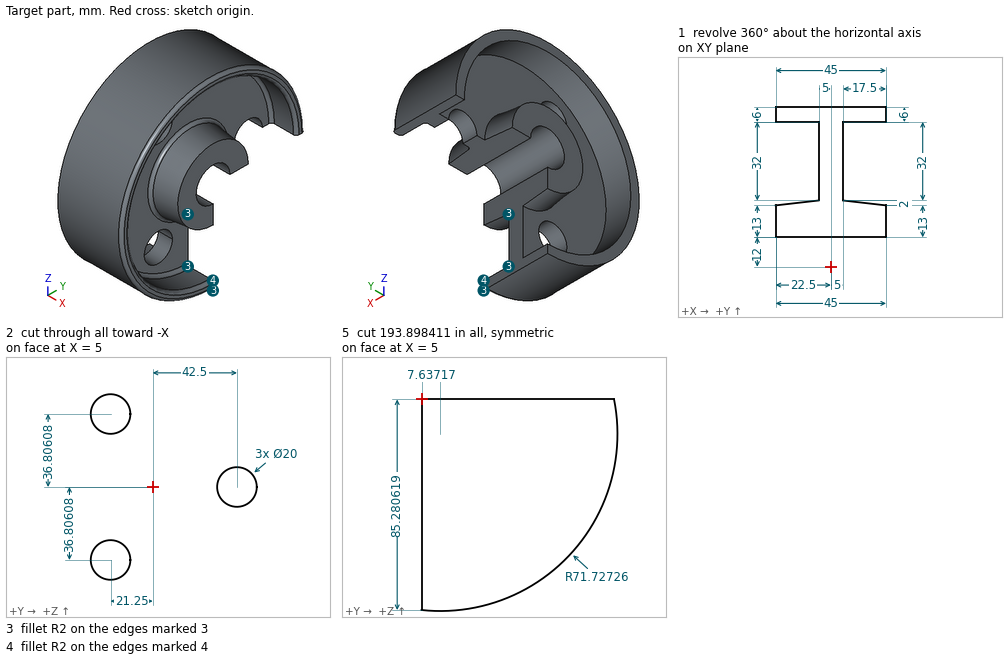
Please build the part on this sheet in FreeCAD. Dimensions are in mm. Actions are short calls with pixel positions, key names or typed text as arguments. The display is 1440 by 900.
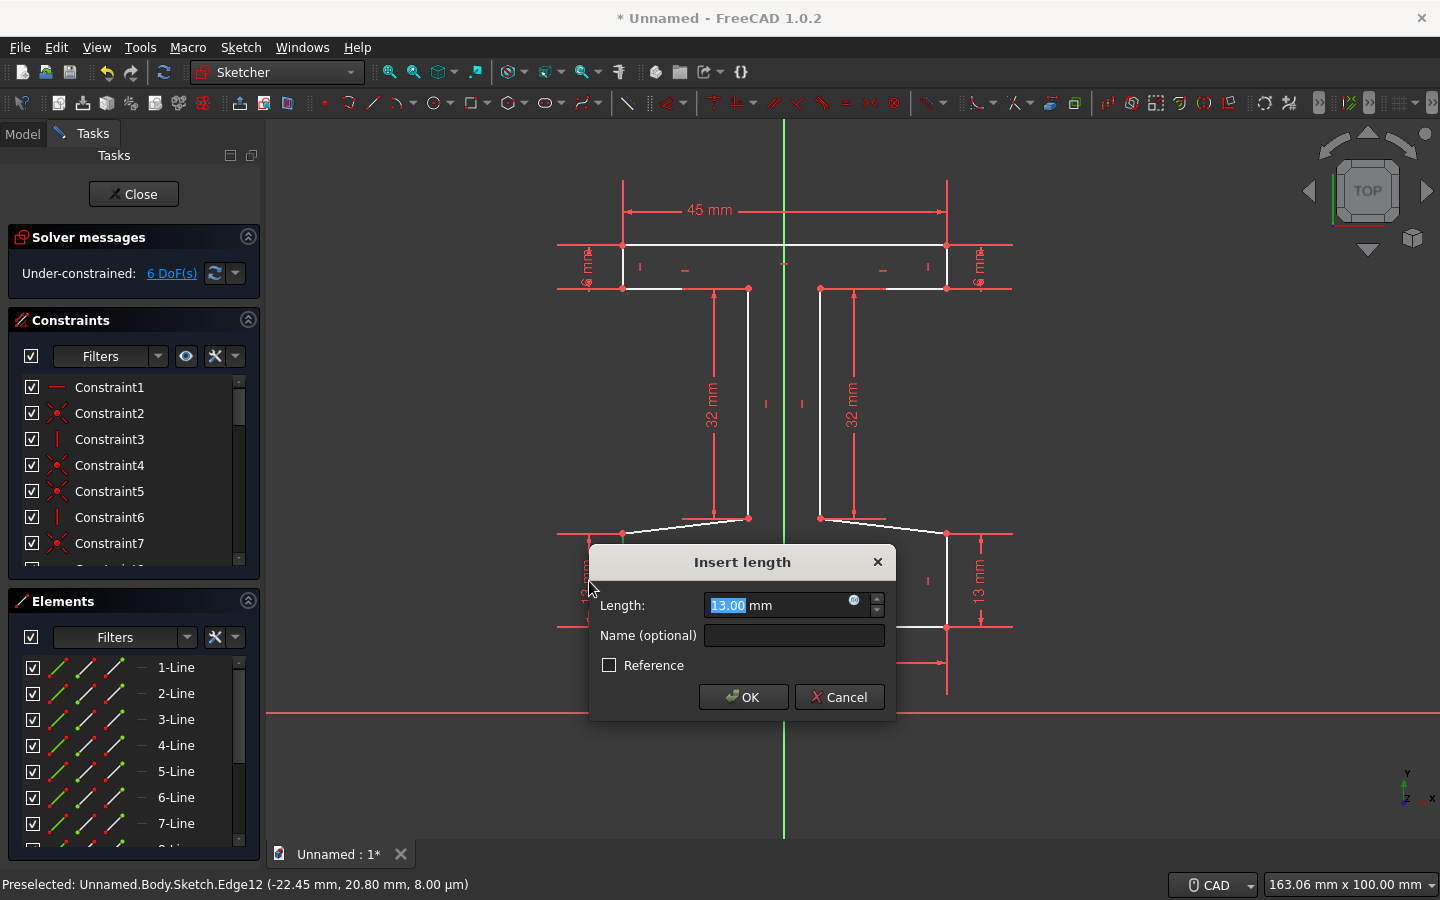
text(13)
key(Return)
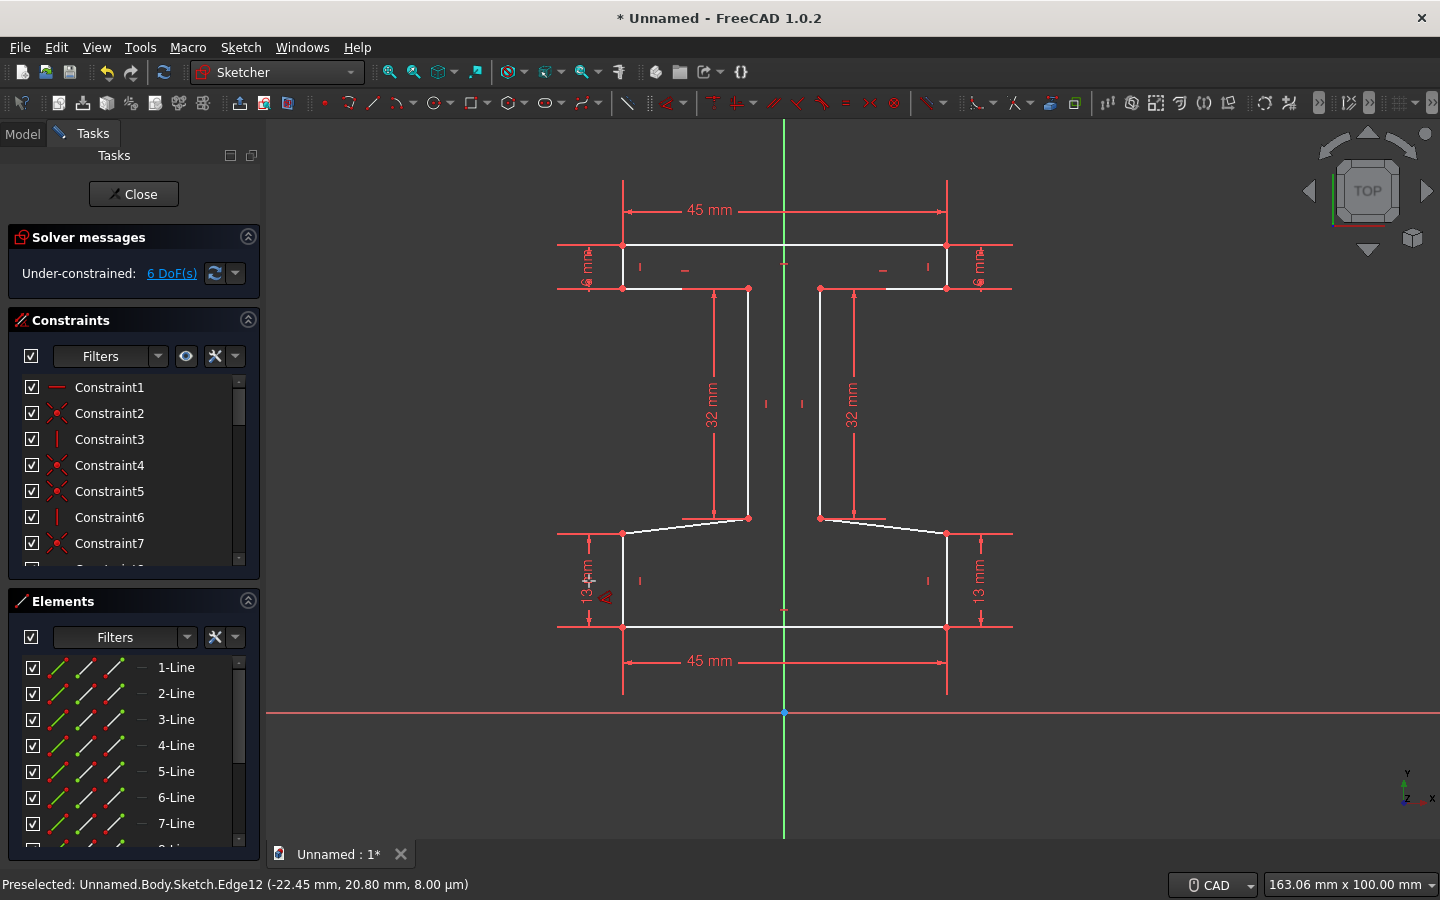
click(820, 519)
click(802, 747)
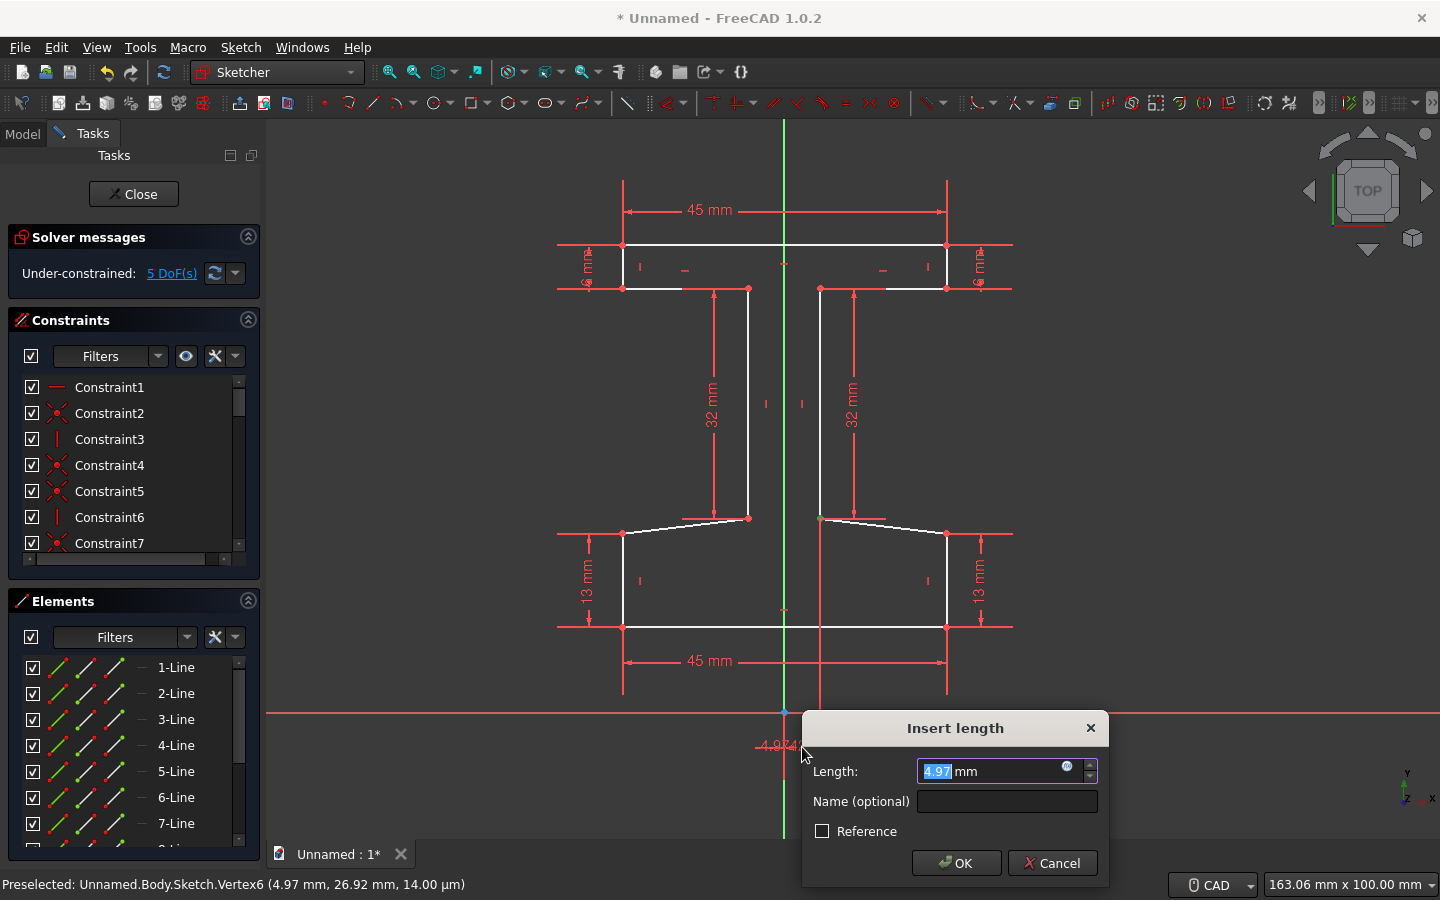
text(5)
key(Return)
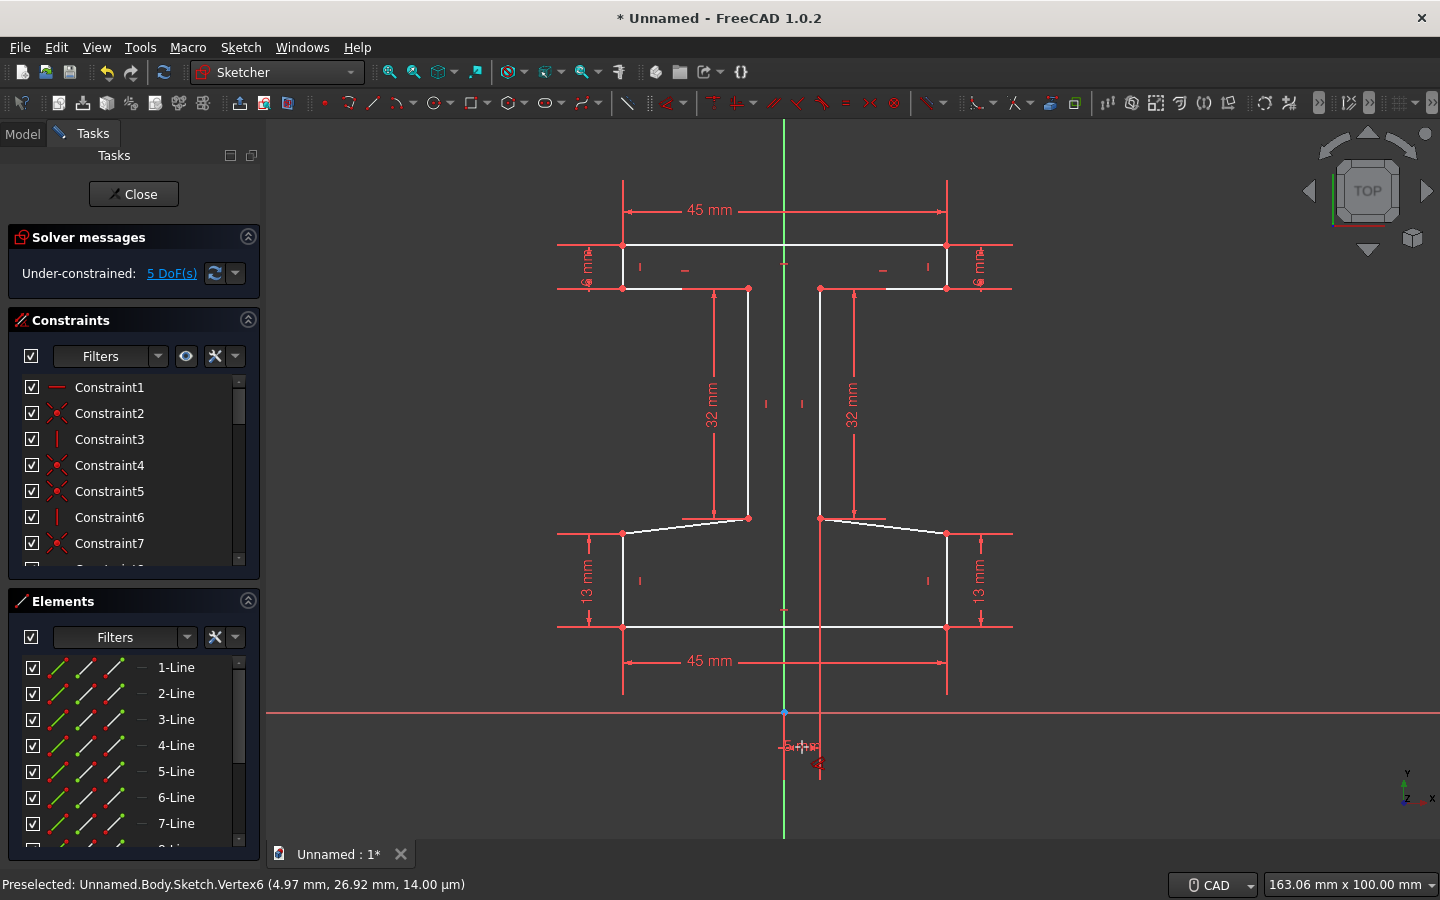
click(748, 289)
click(766, 771)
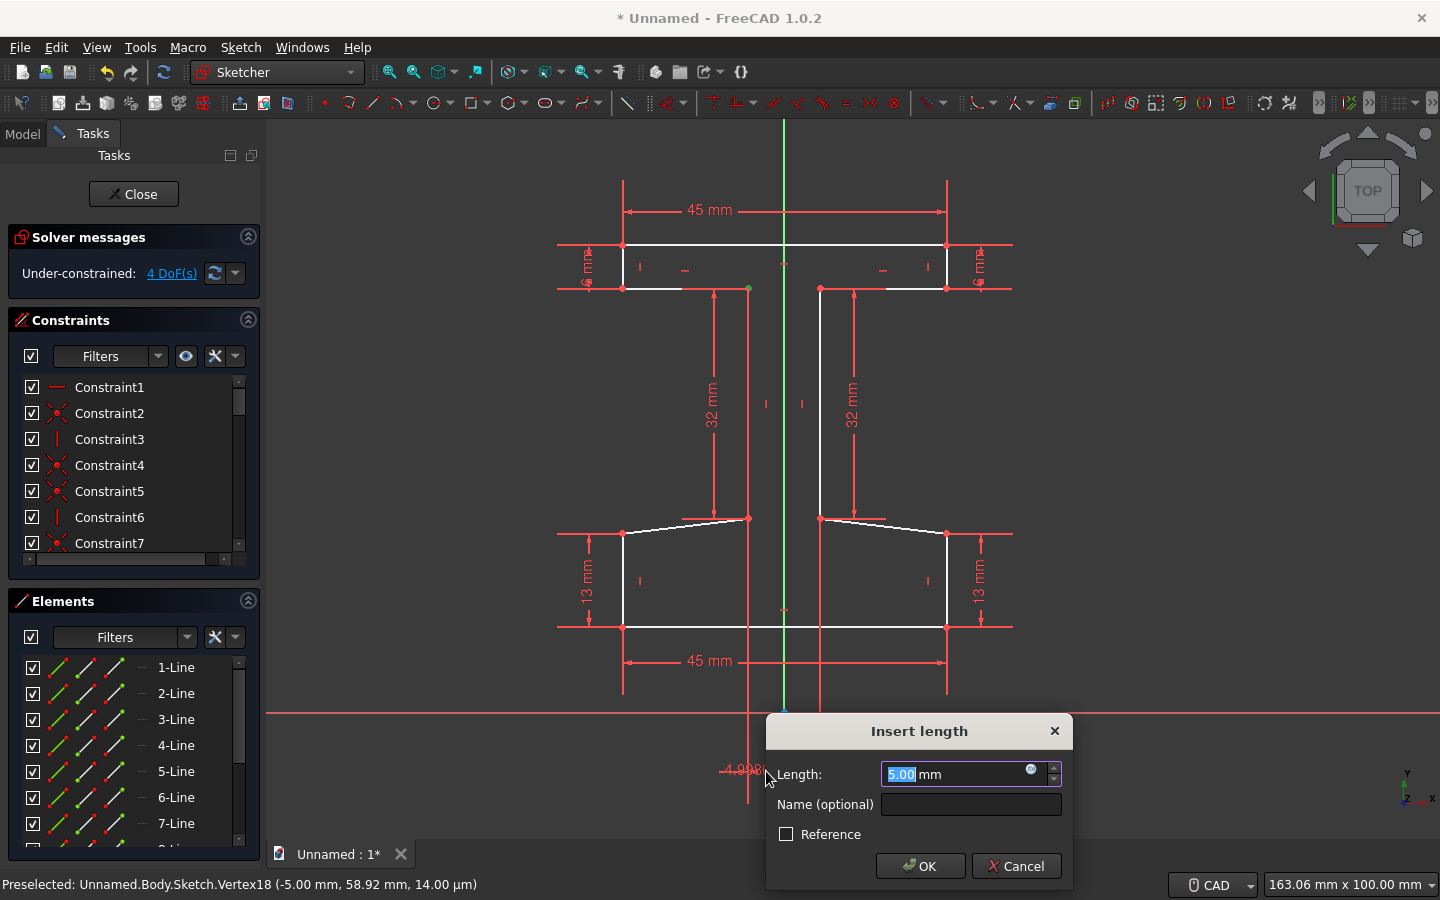
text(5)
key(Return)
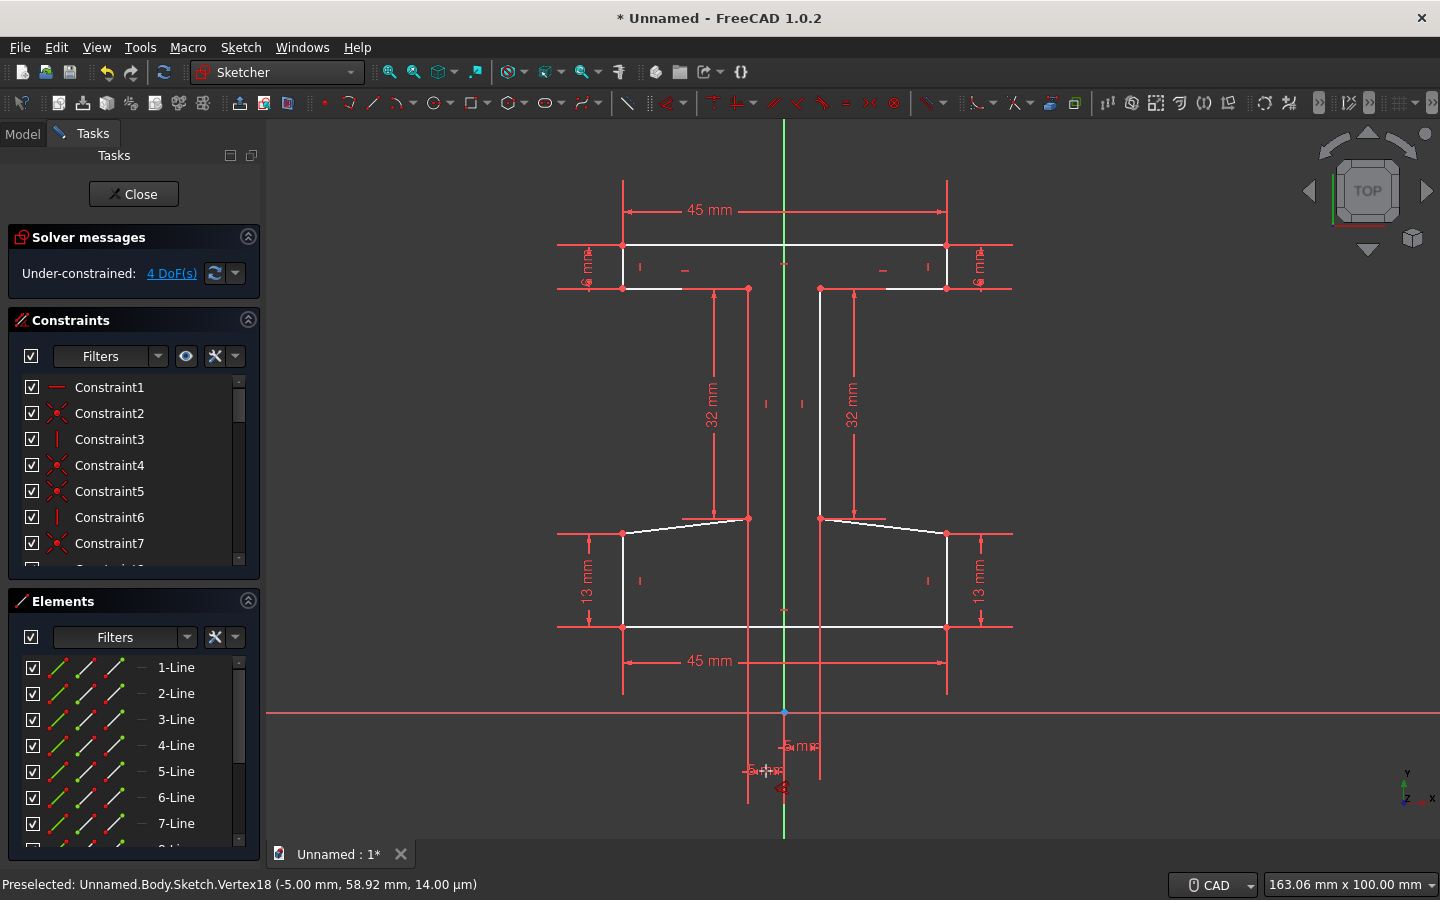
scroll(909, 529, up, 6)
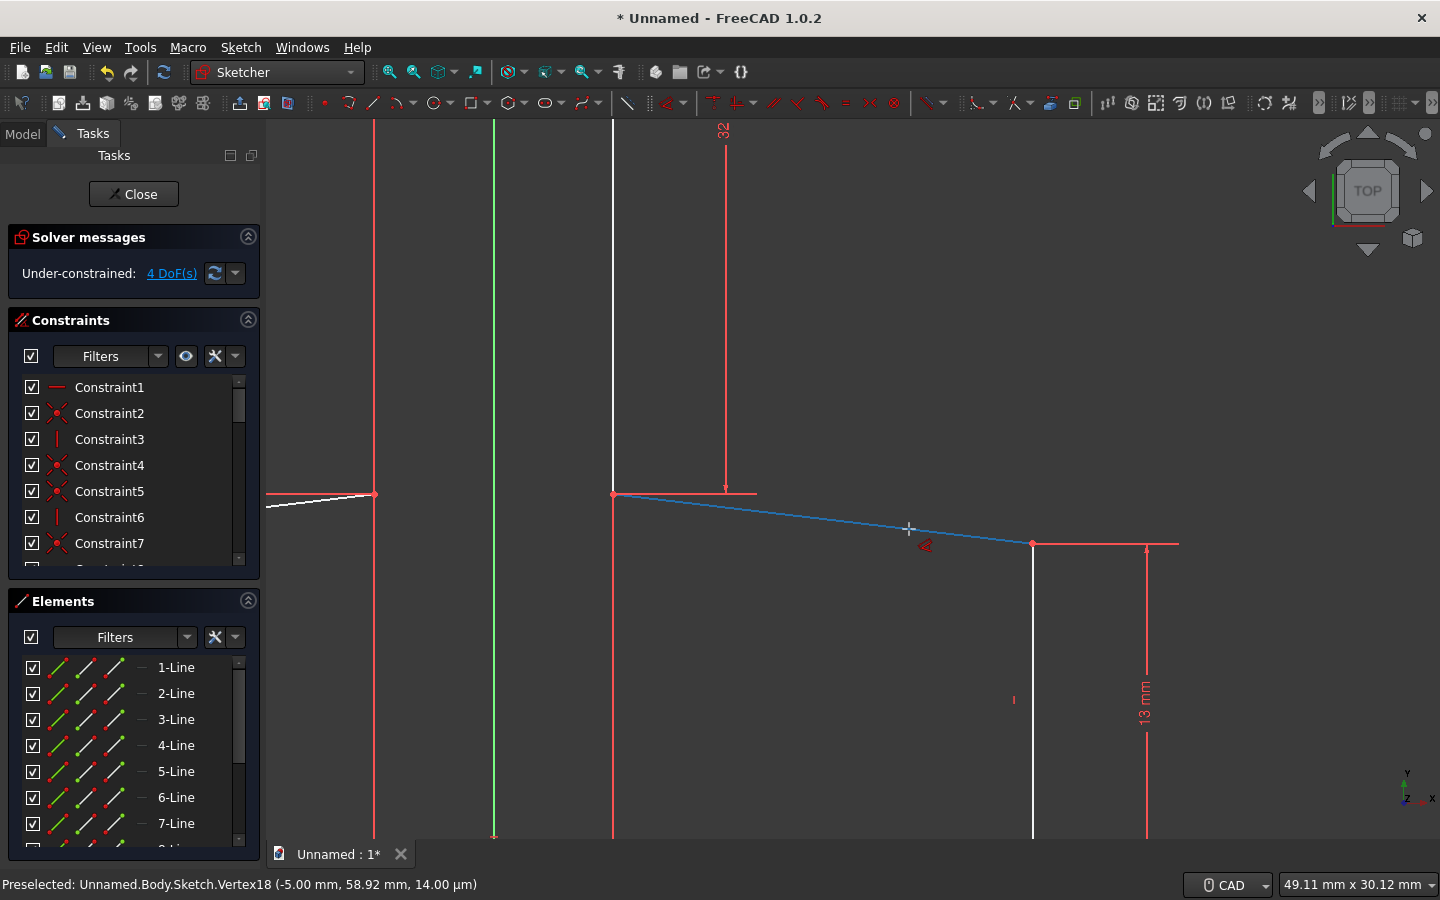
click(907, 529)
click(1067, 519)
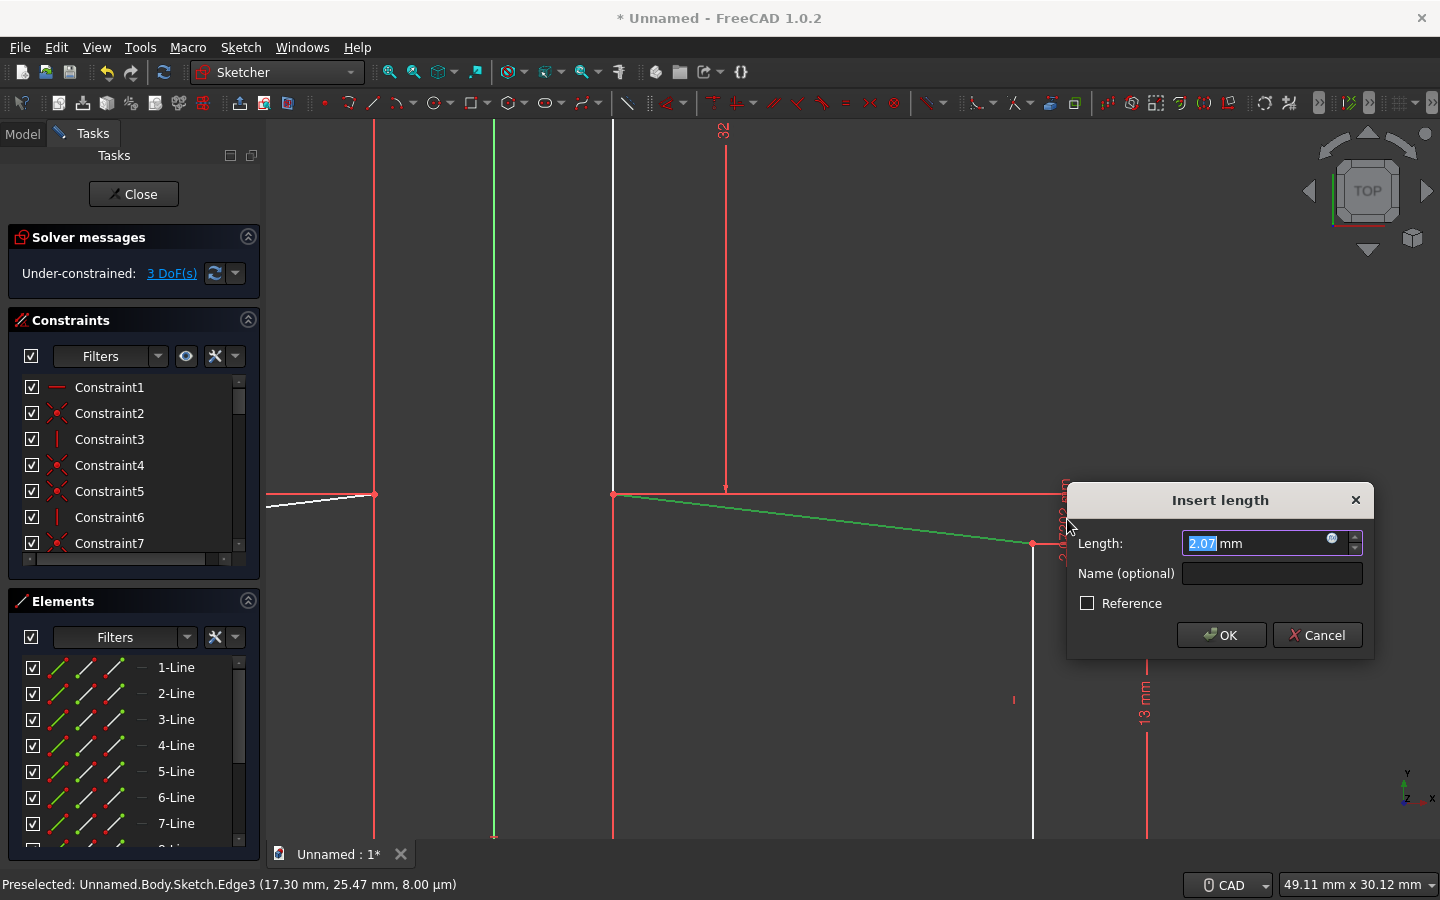
text(2)
key(Return)